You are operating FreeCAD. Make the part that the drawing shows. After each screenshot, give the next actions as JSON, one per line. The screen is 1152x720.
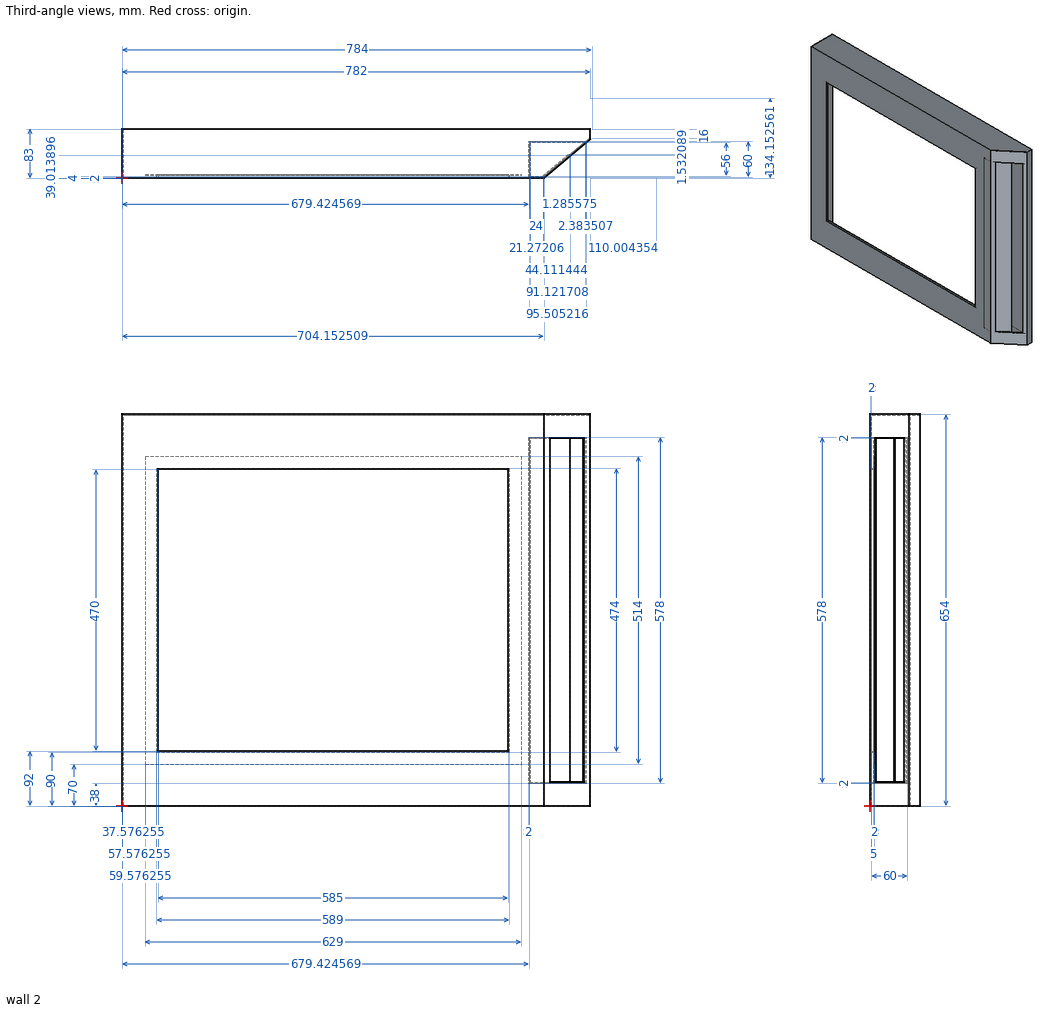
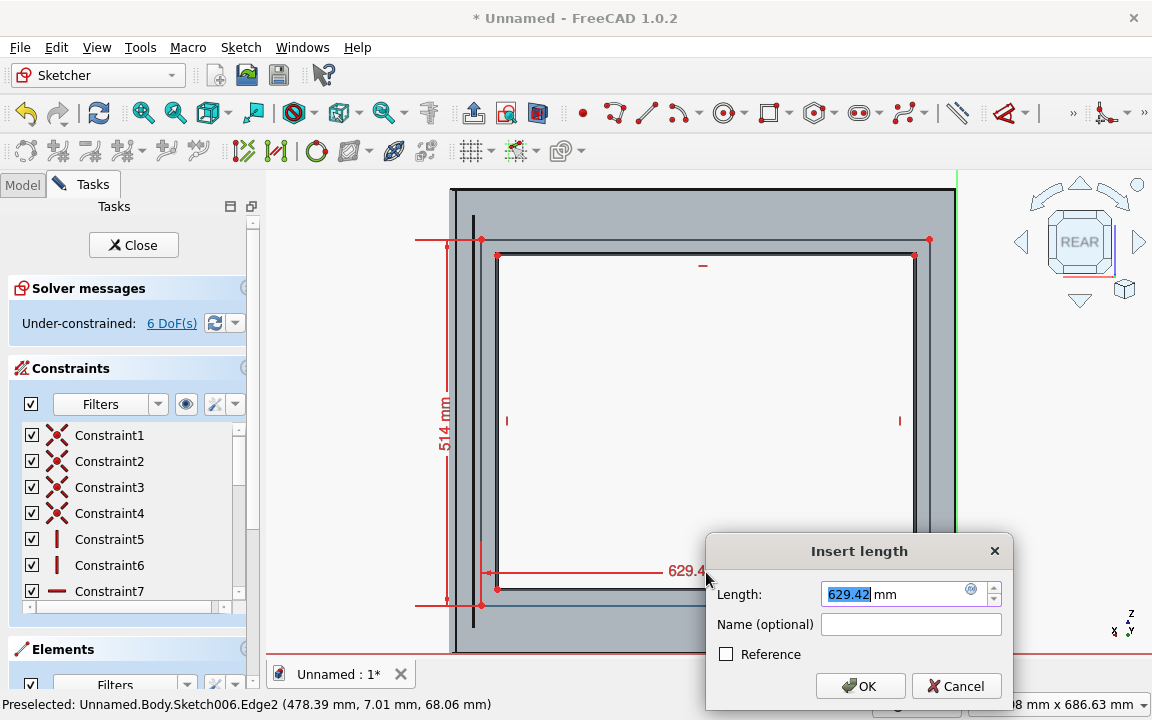
{"action": "type", "text": "629"}
{"action": "key", "text": "Return"}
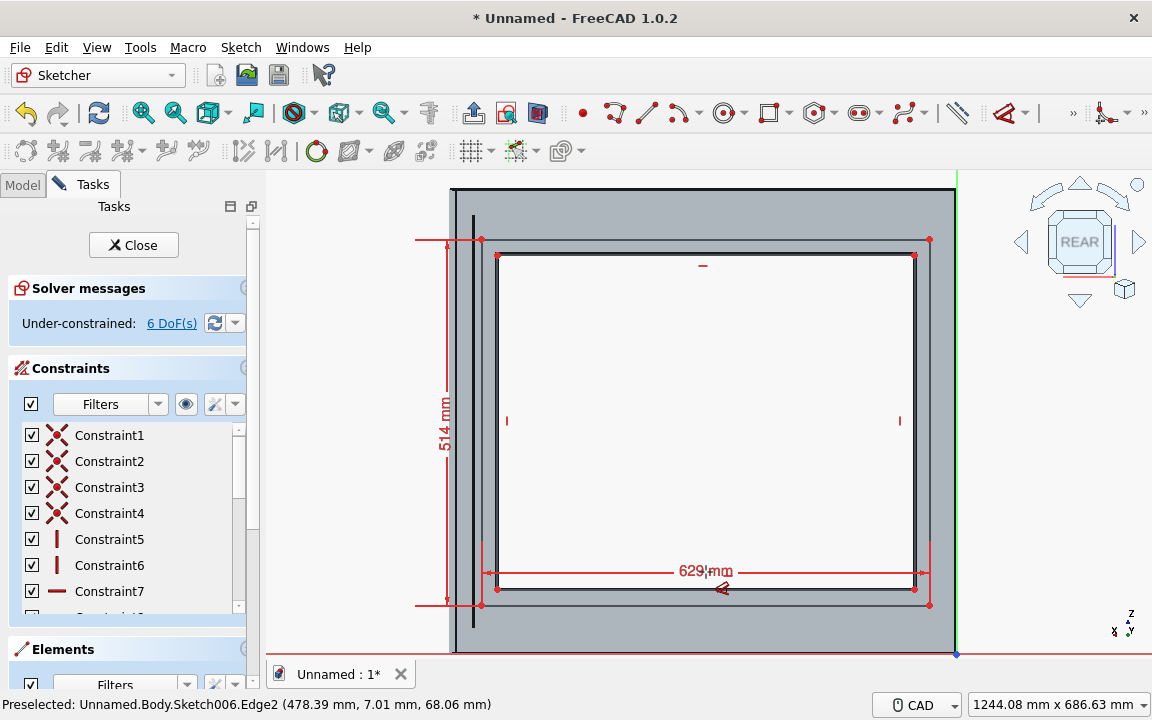
{"action": "left_click", "coordinate": [497, 356]}
{"action": "left_click", "coordinate": [463, 346]}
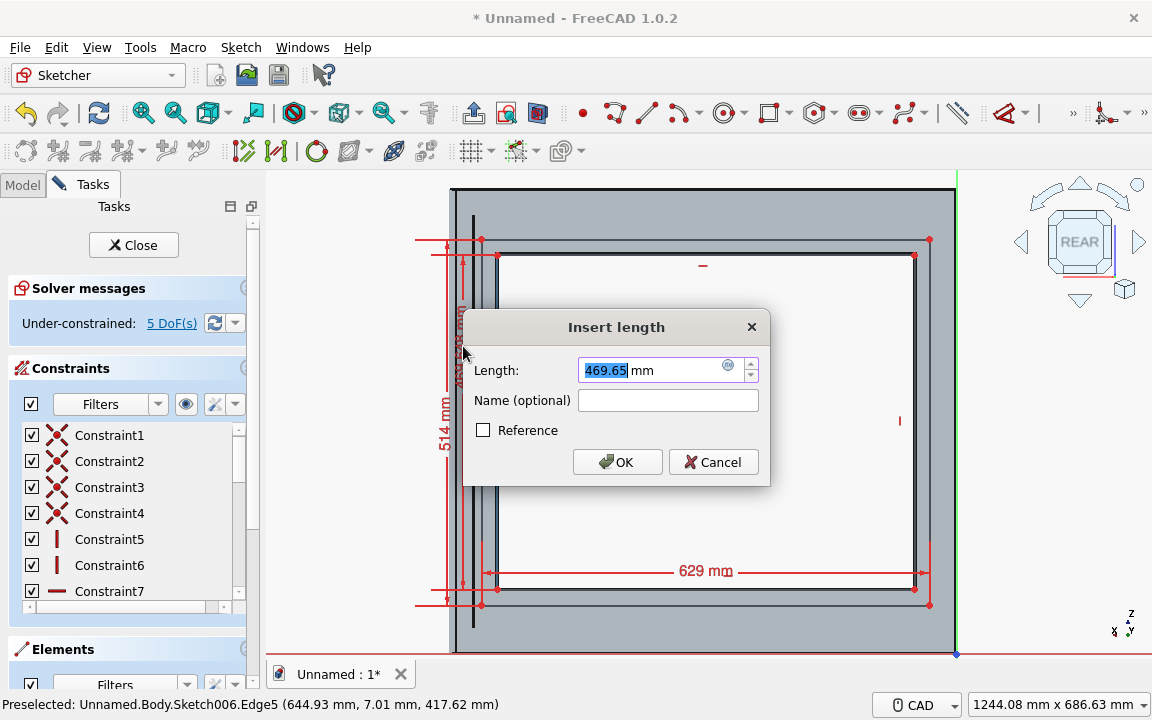
{"action": "type", "text": "470"}
{"action": "key", "text": "Return"}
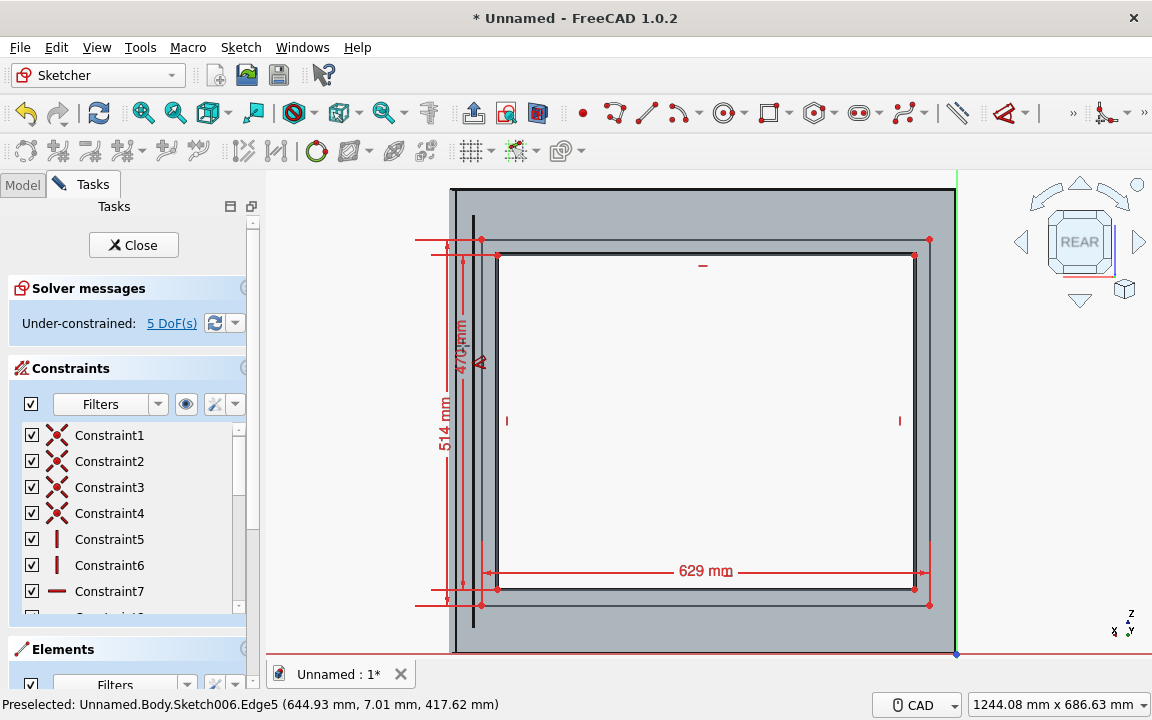
{"action": "left_click", "coordinate": [623, 590]}
{"action": "left_click", "coordinate": [706, 624]}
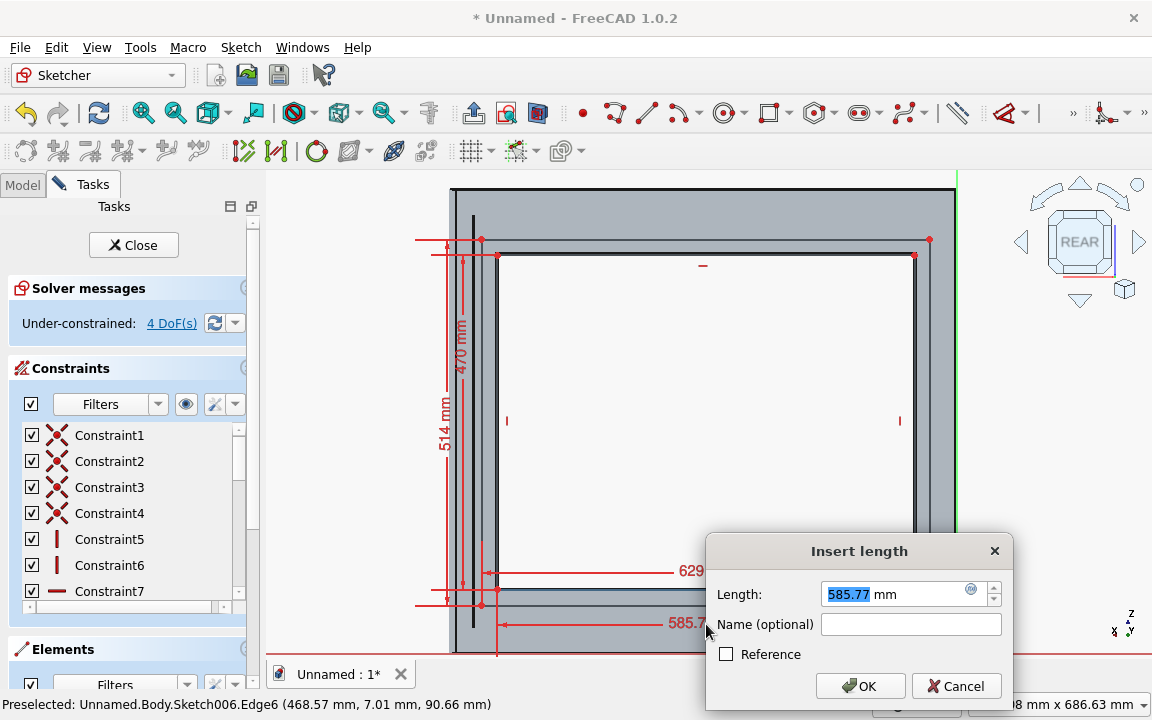
{"action": "type", "text": "585"}
{"action": "key", "text": "Return"}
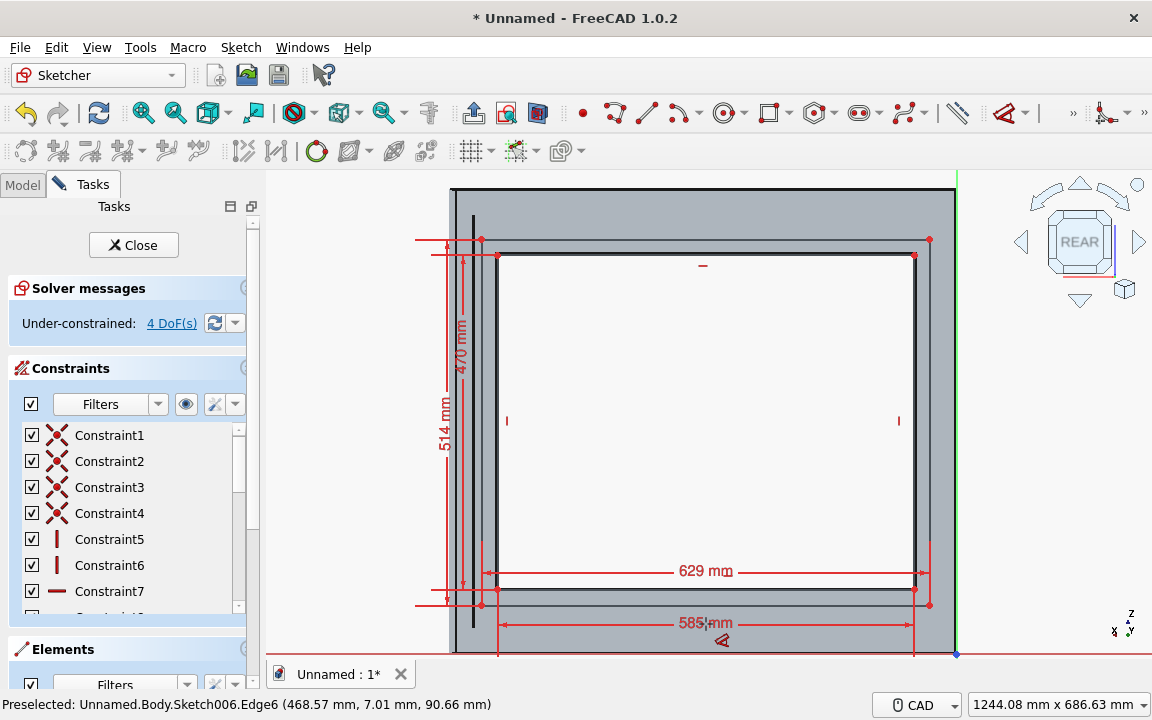
{"action": "left_click", "coordinate": [482, 606]}
{"action": "left_click", "coordinate": [448, 618]}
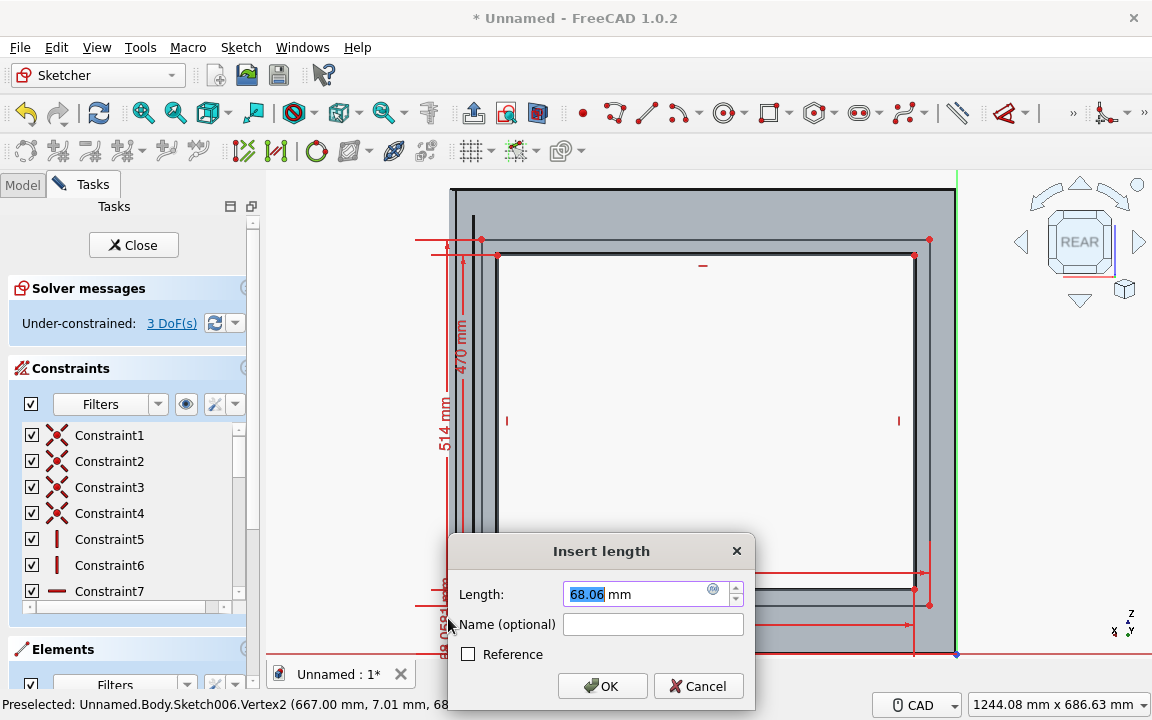
{"action": "type", "text": "70"}
{"action": "key", "text": "Return"}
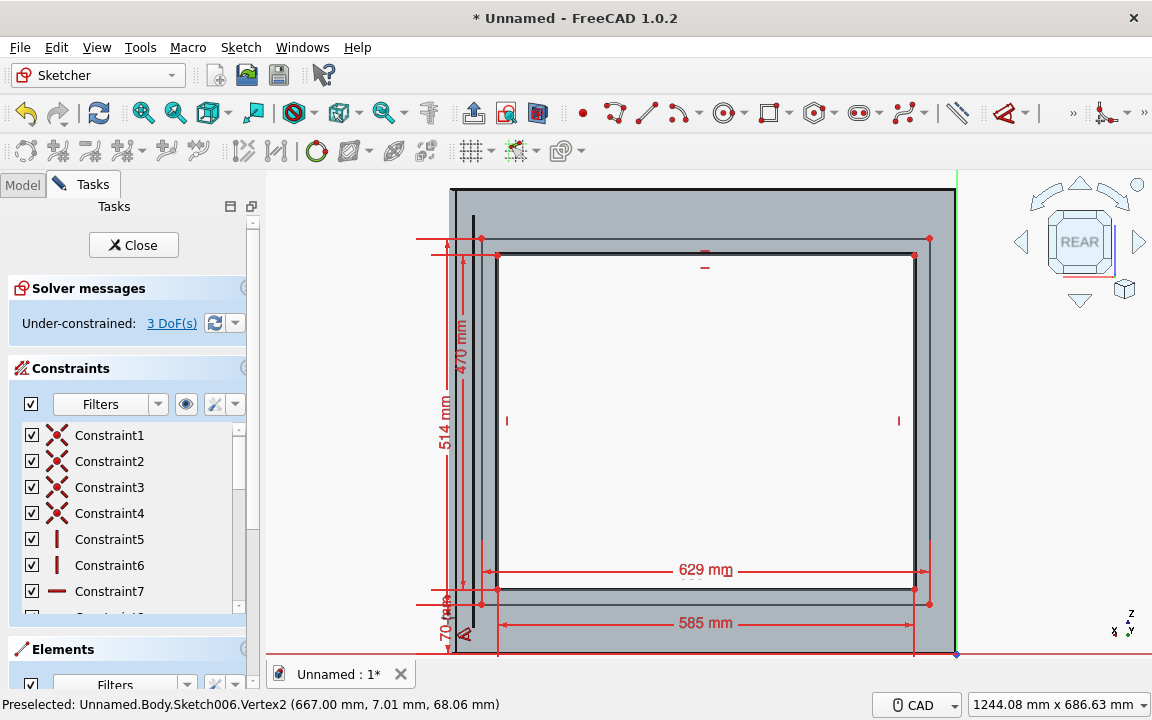
{"action": "left_click", "coordinate": [498, 590]}
{"action": "left_click", "coordinate": [464, 596]}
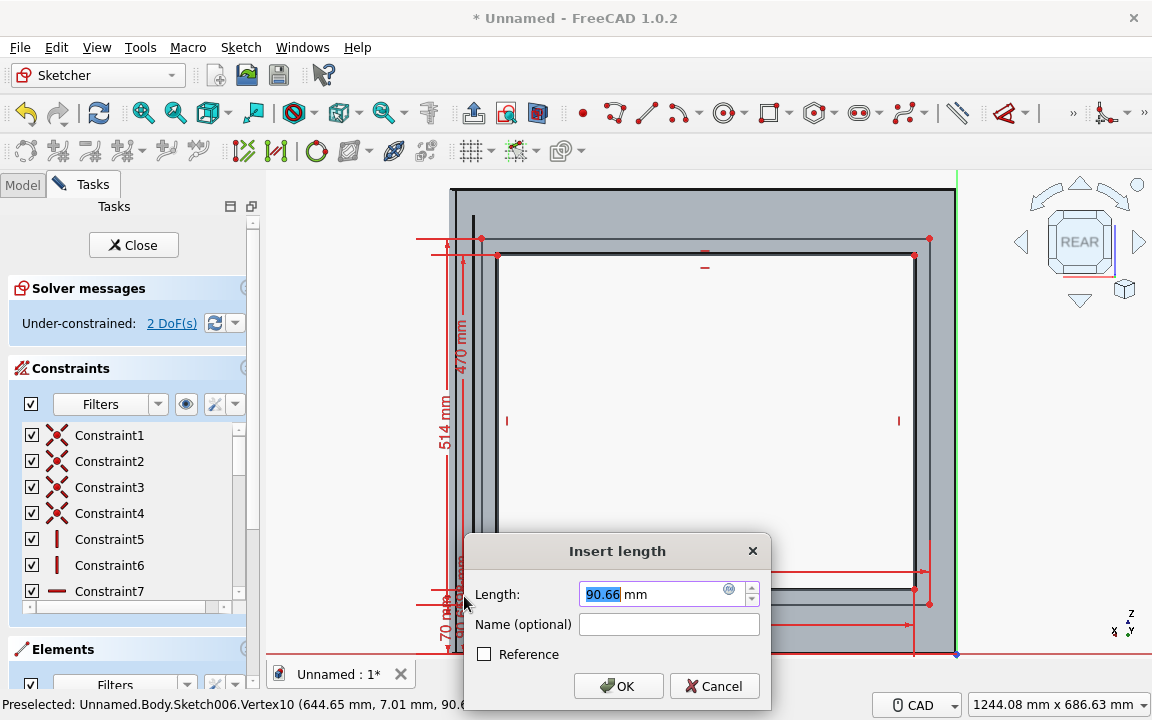
{"action": "type", "text": "92"}
{"action": "key", "text": "Return"}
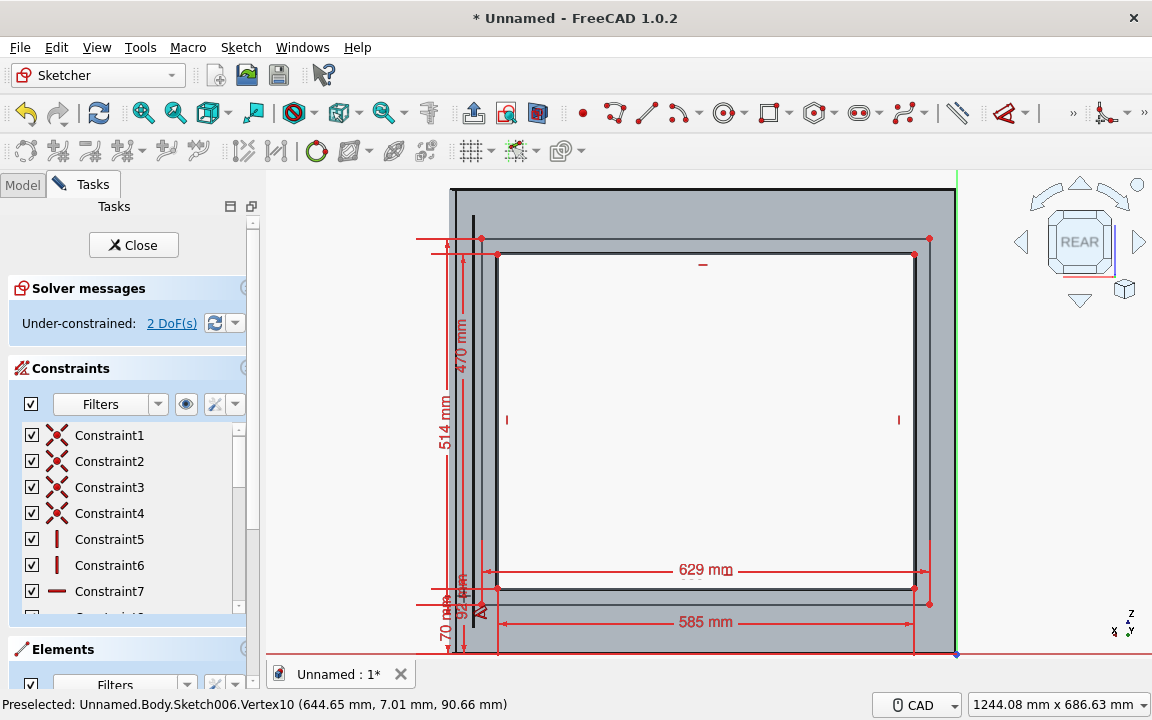
{"action": "scroll", "coordinate": [930, 605], "scroll_direction": "up", "scroll_amount": 2}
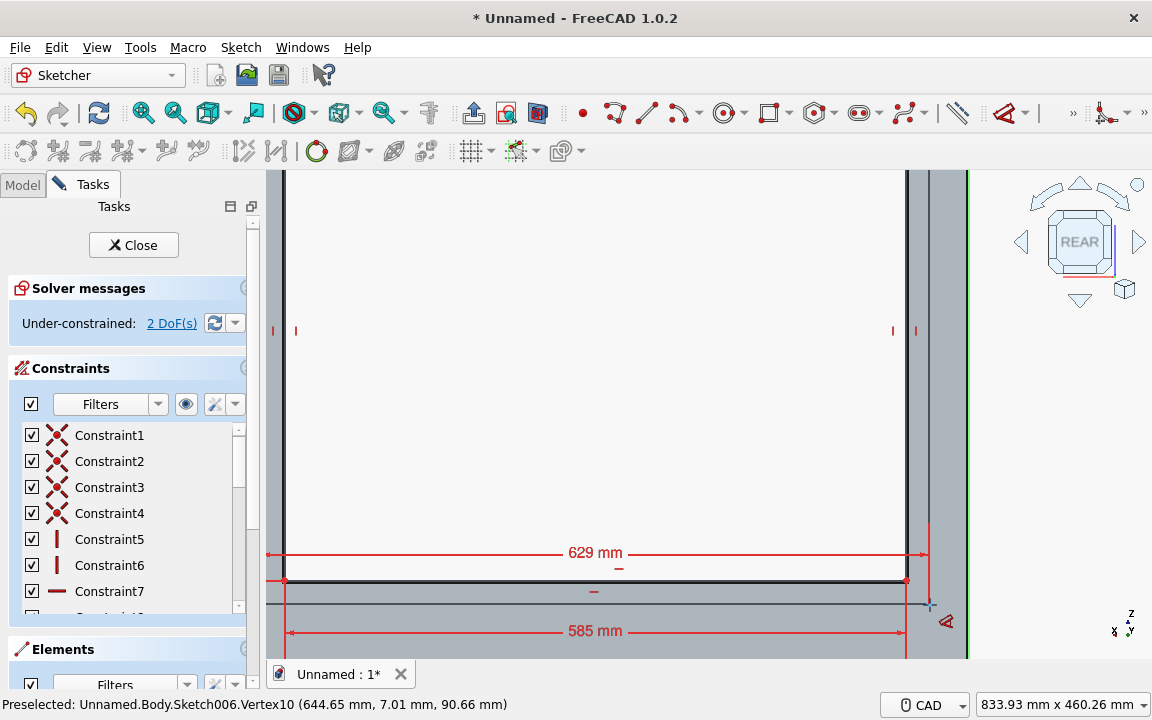
{"action": "left_click", "coordinate": [929, 604]}
{"action": "left_click", "coordinate": [949, 570]}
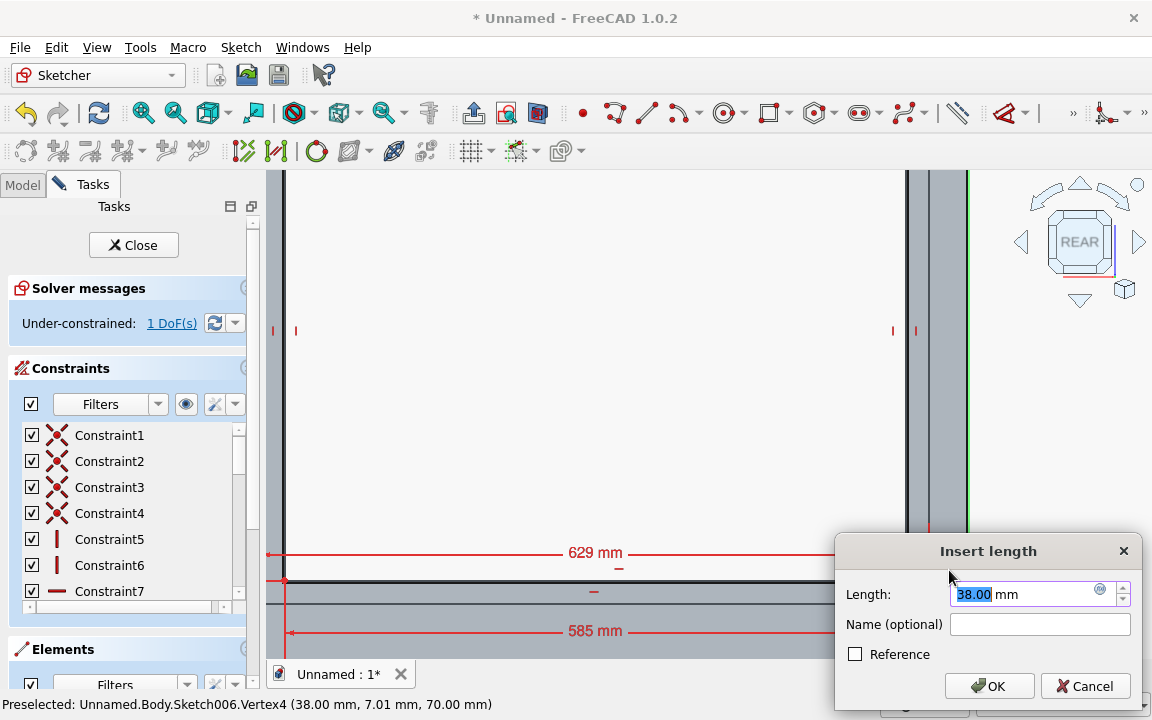
{"action": "type", "text": "37.576255"}
{"action": "key", "text": "Return"}